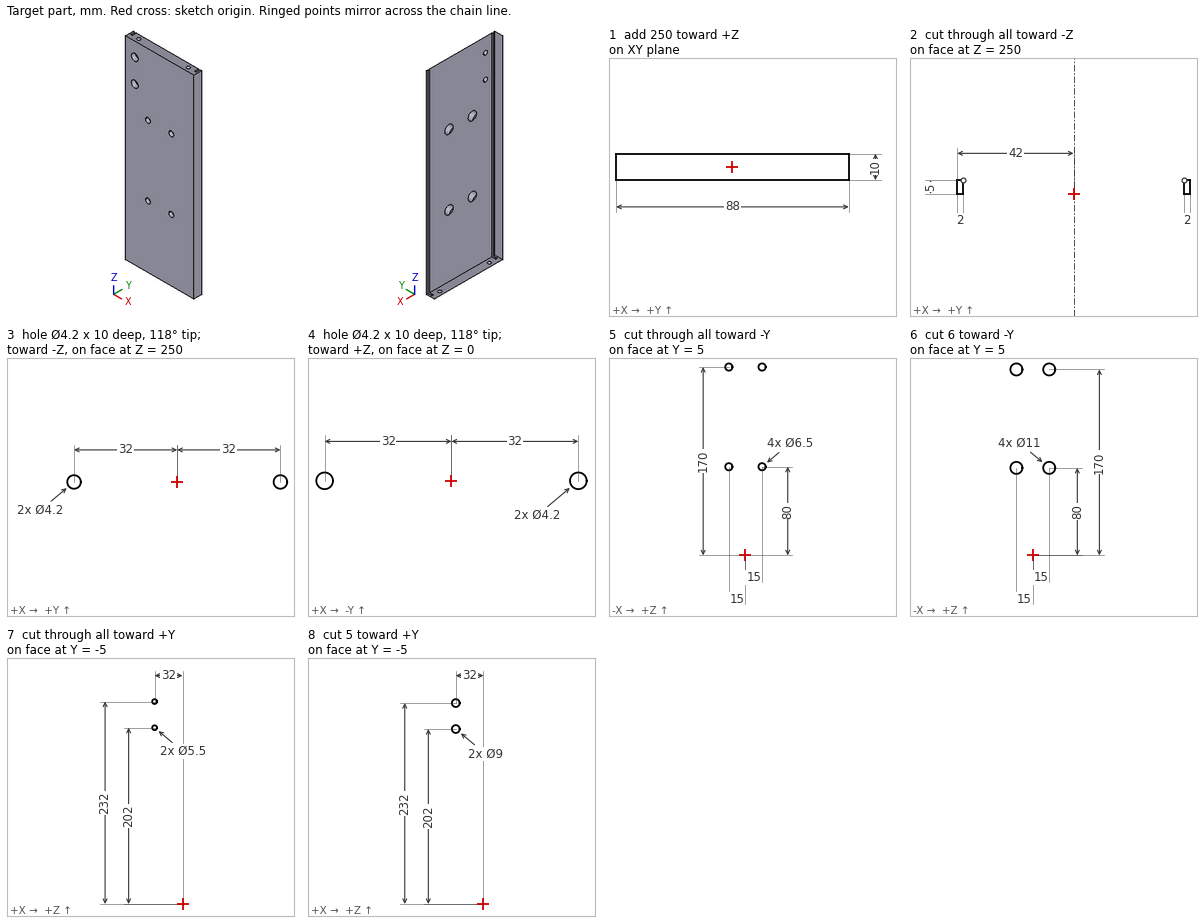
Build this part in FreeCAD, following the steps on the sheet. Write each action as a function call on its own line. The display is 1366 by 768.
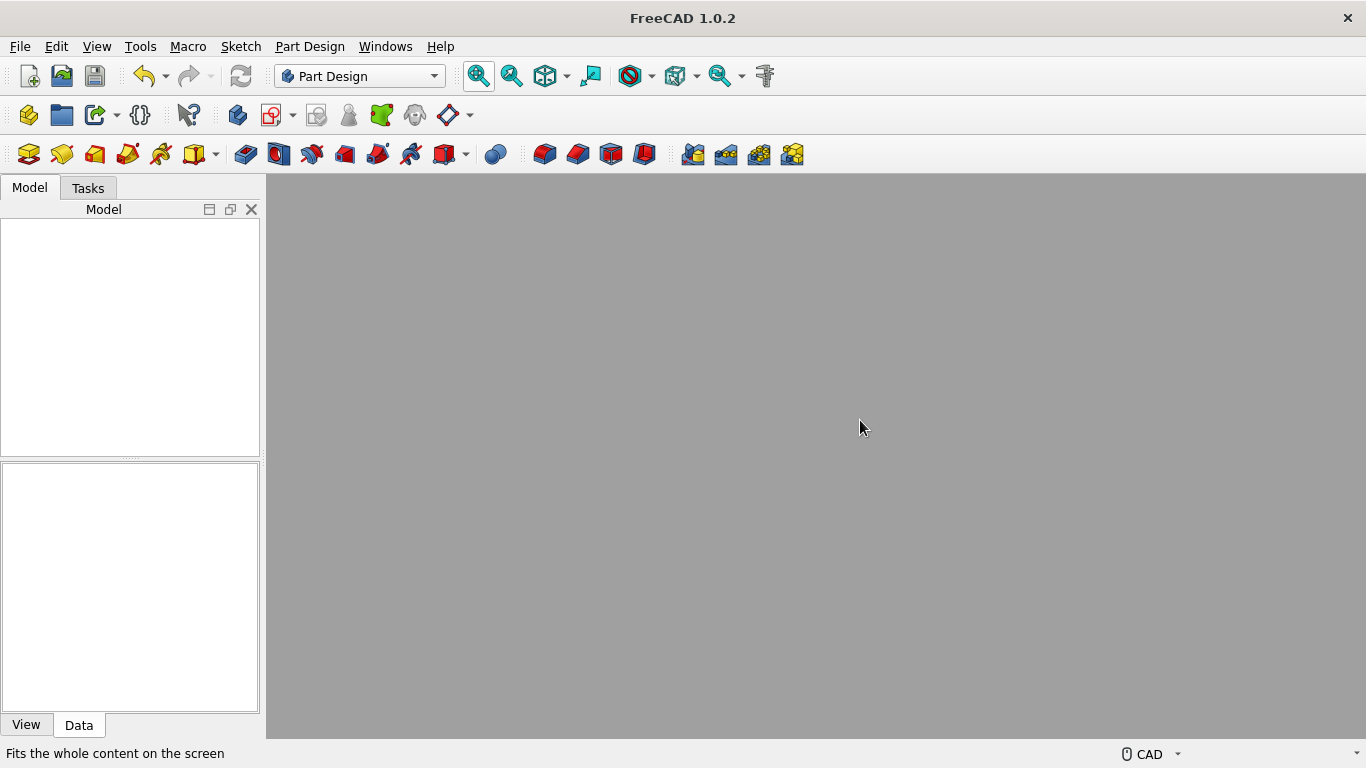
click(29, 76)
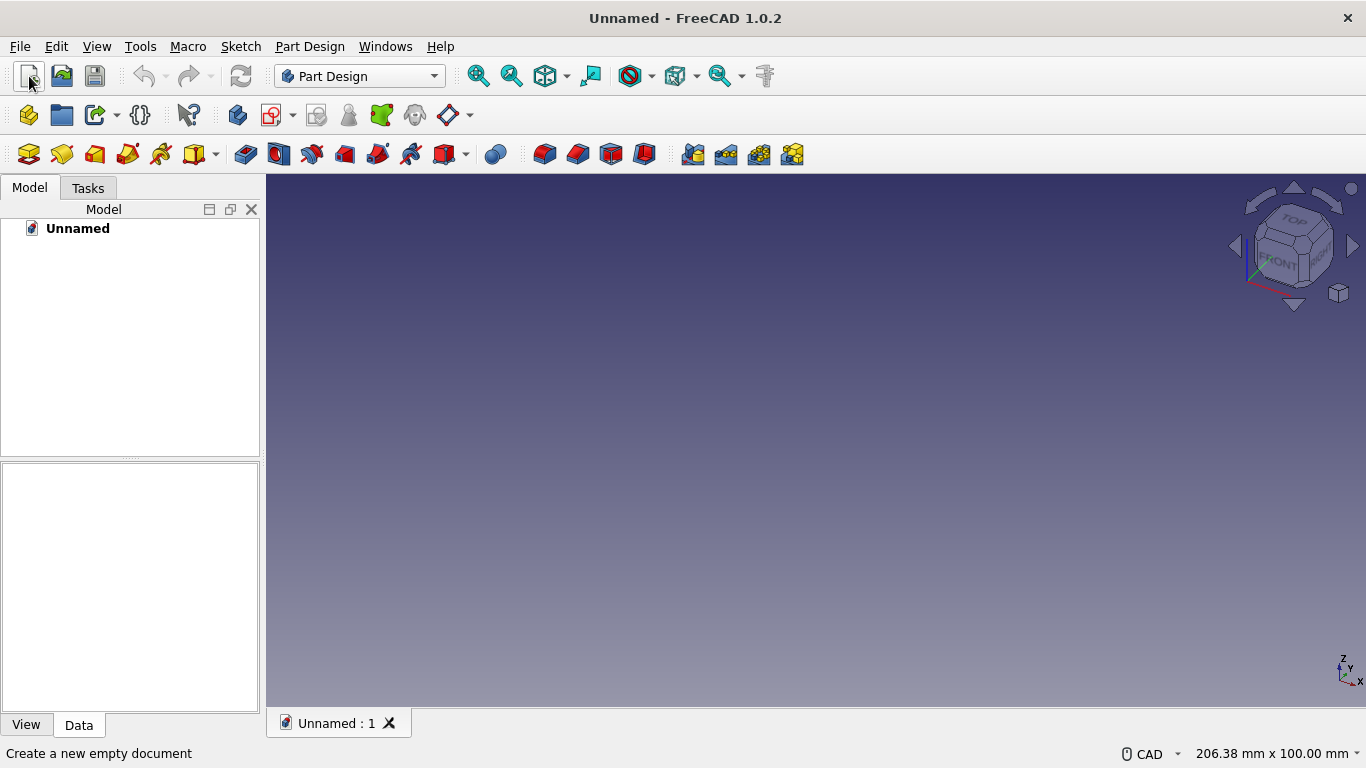
click(270, 116)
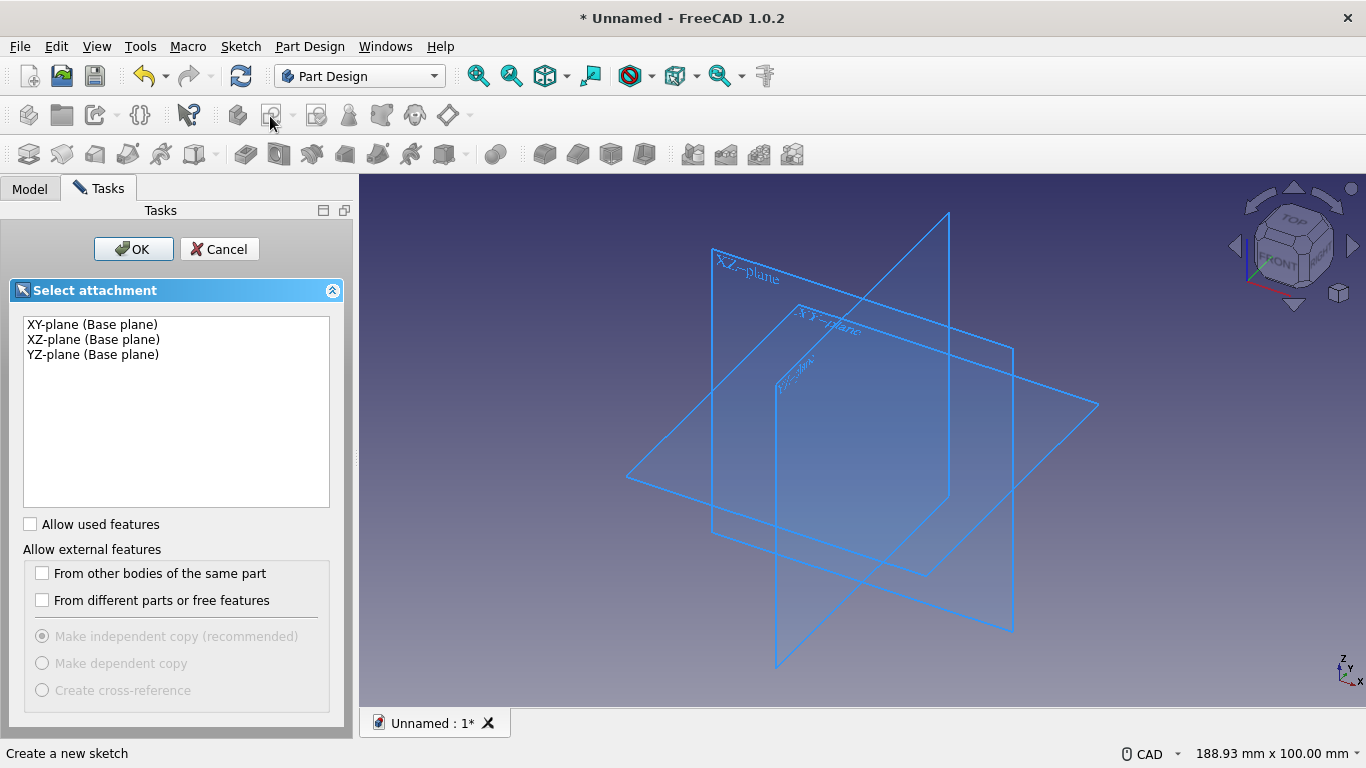
click(84, 324)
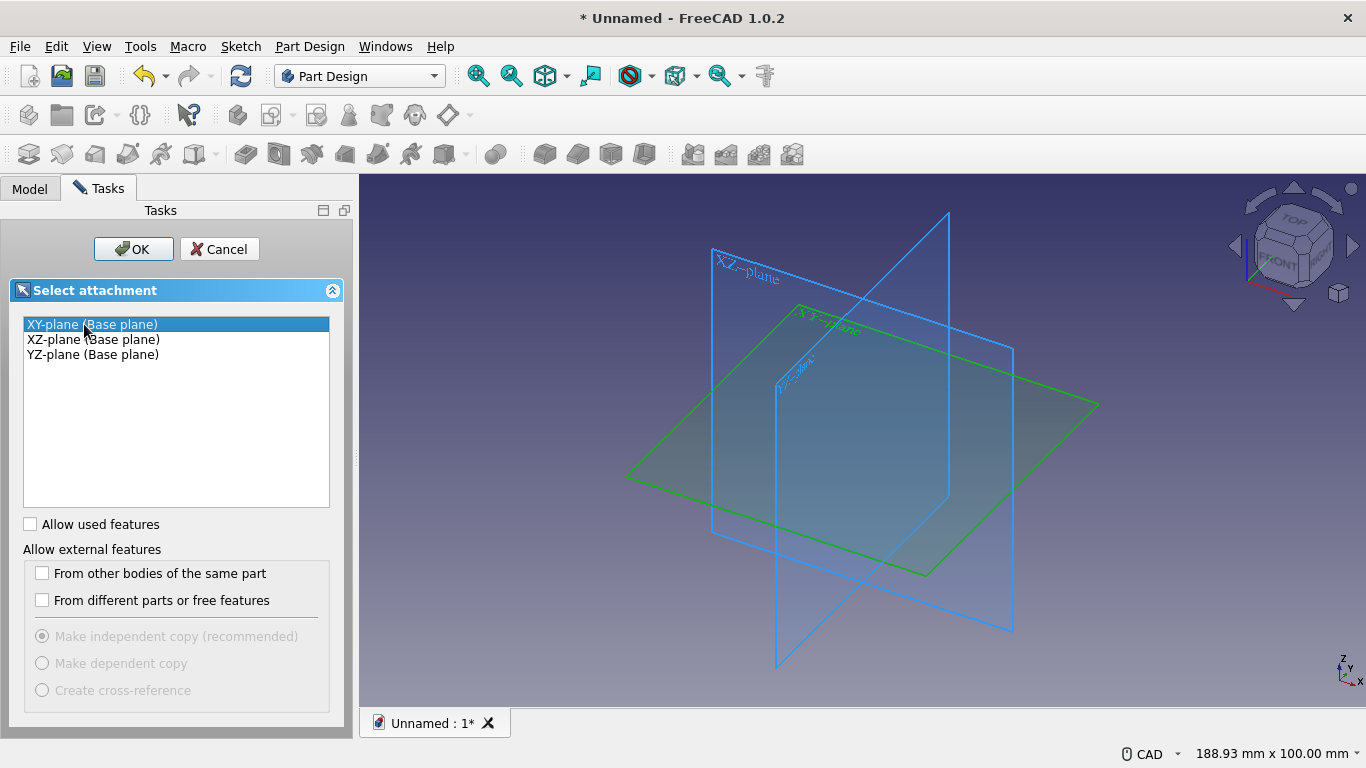
click(134, 249)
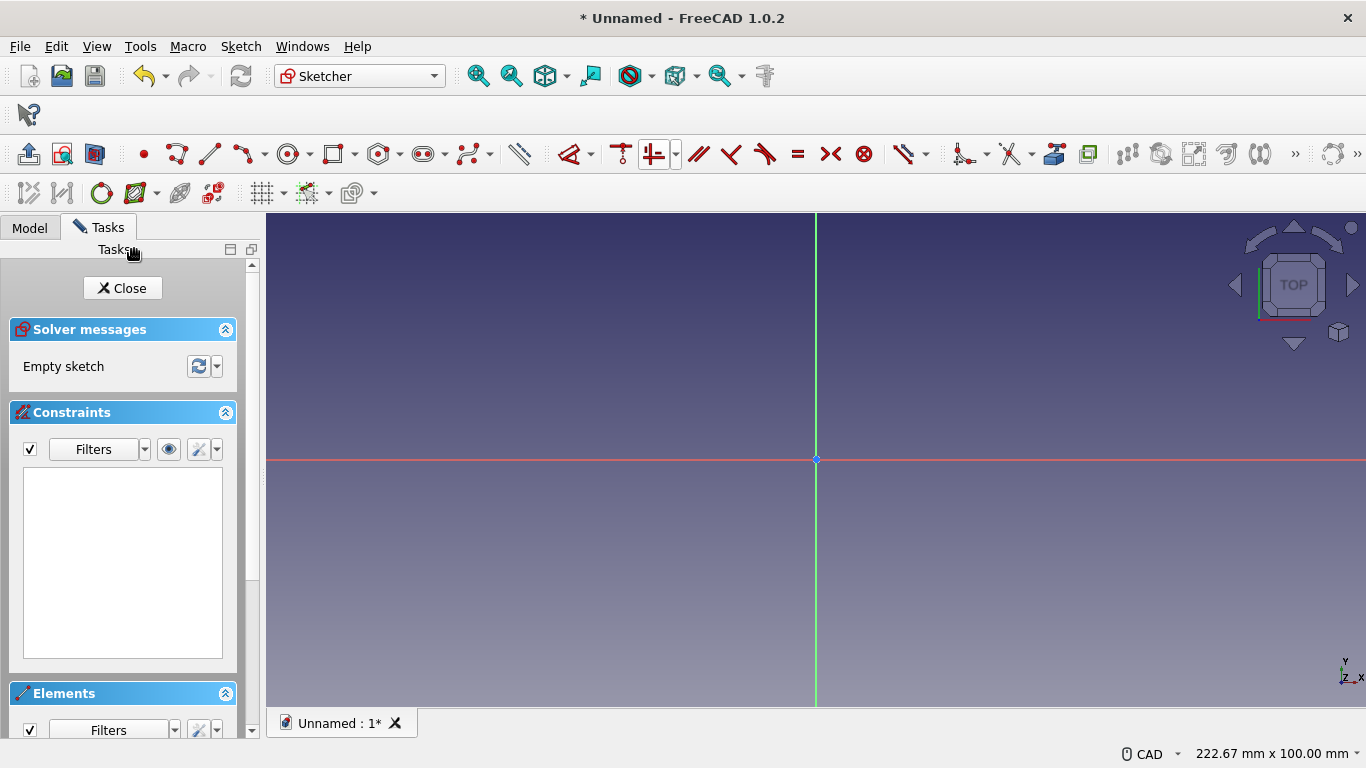
scroll(955, 460, up, 2)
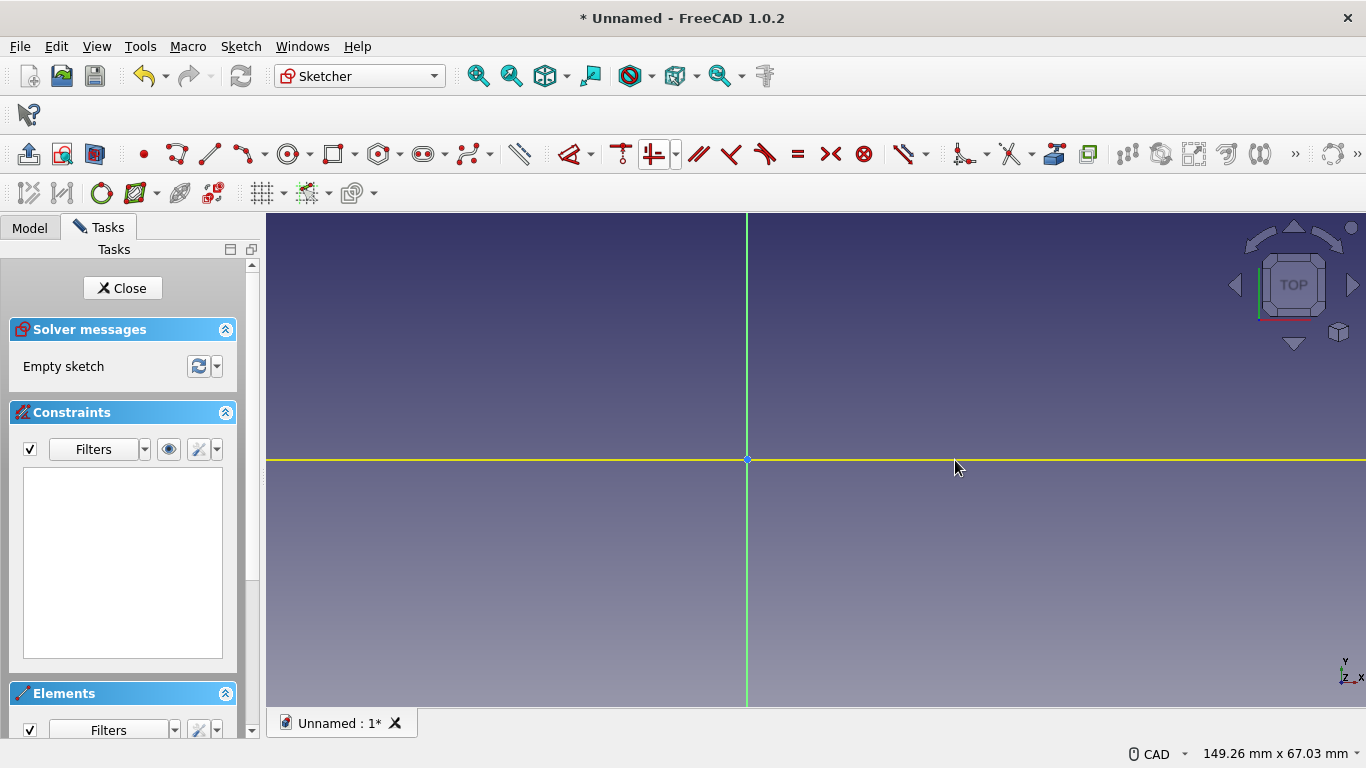
key(g)
key(v)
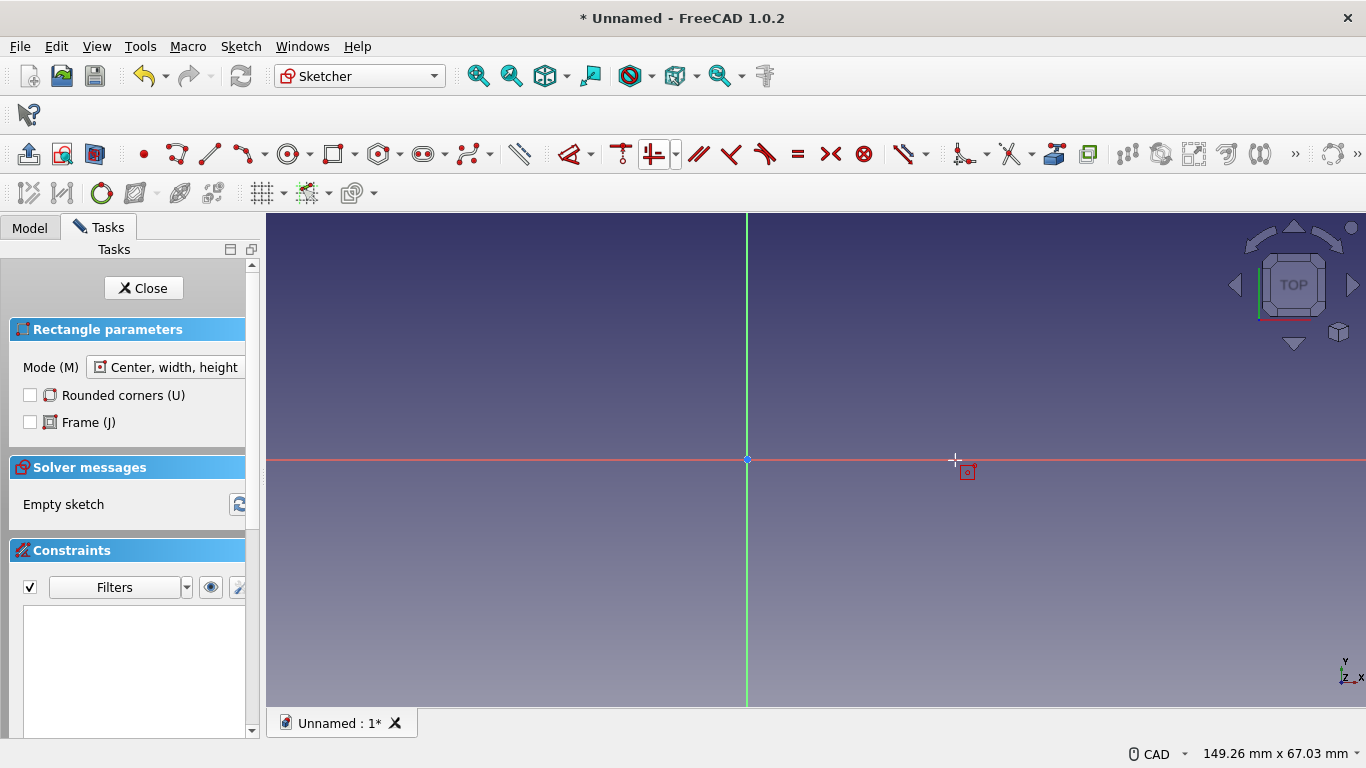
click(747, 460)
move(1072, 423)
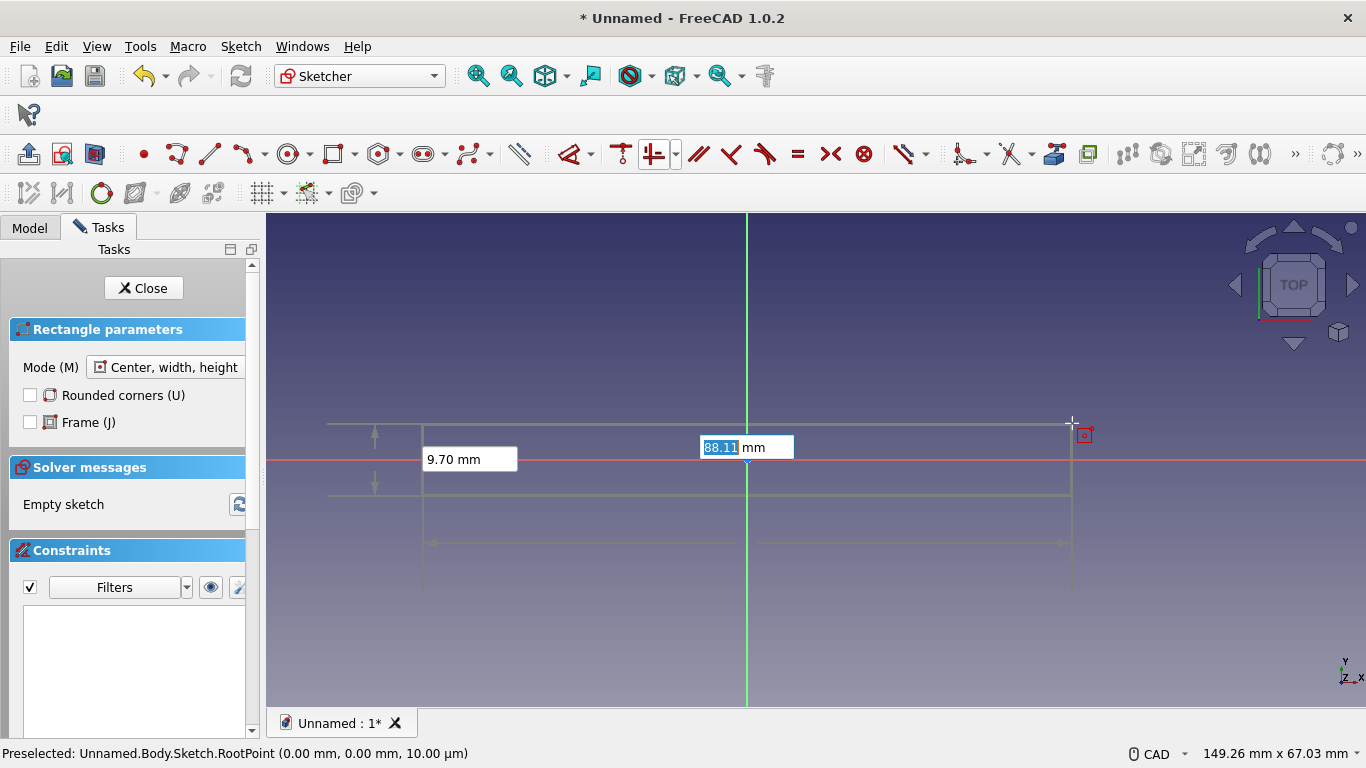
text(88)
key(Tab)
text(10)
key(Return)
key(Escape)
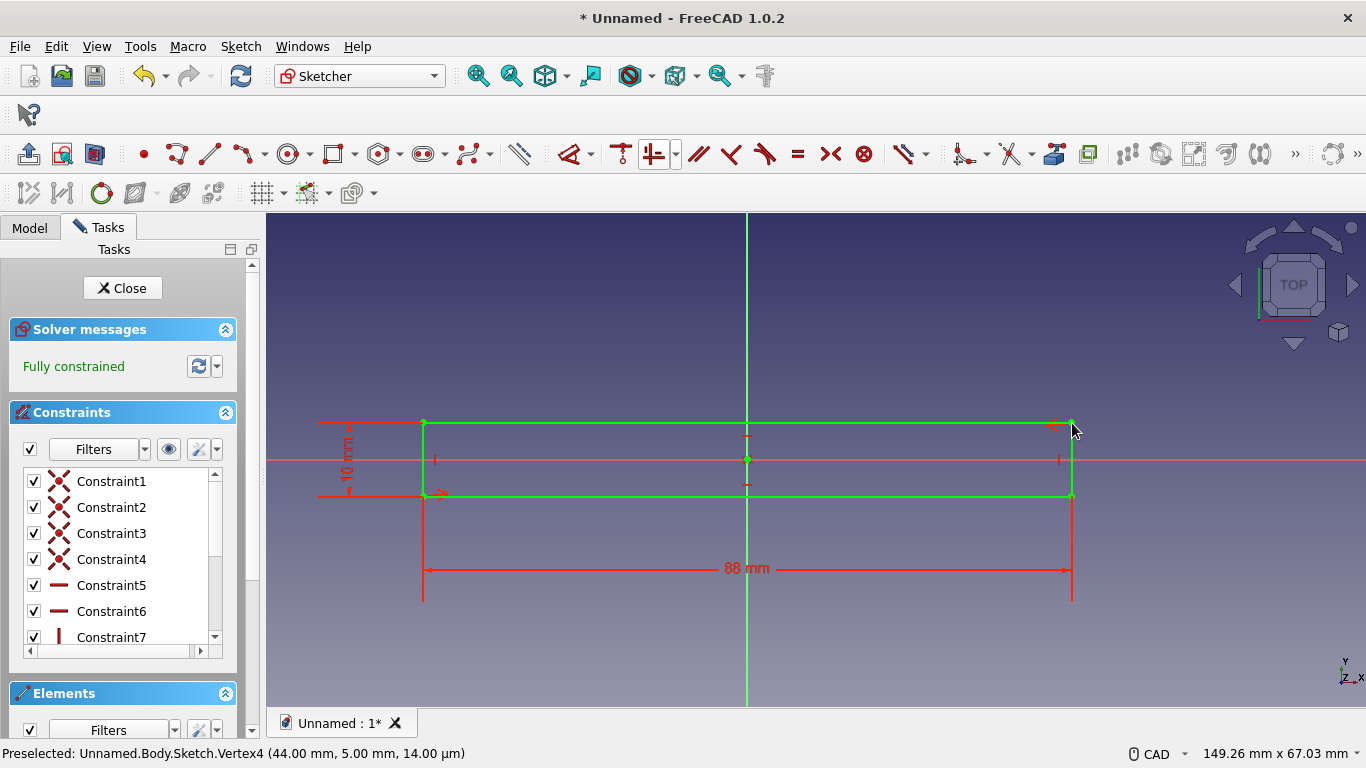
click(123, 288)